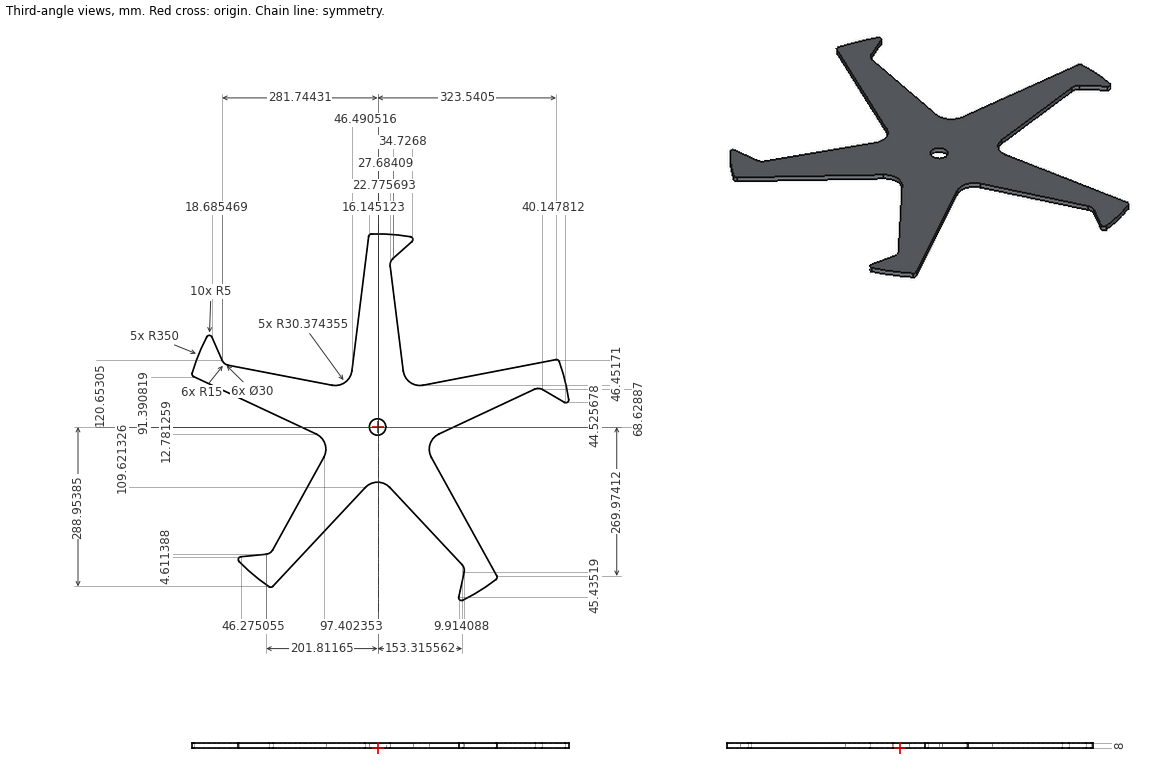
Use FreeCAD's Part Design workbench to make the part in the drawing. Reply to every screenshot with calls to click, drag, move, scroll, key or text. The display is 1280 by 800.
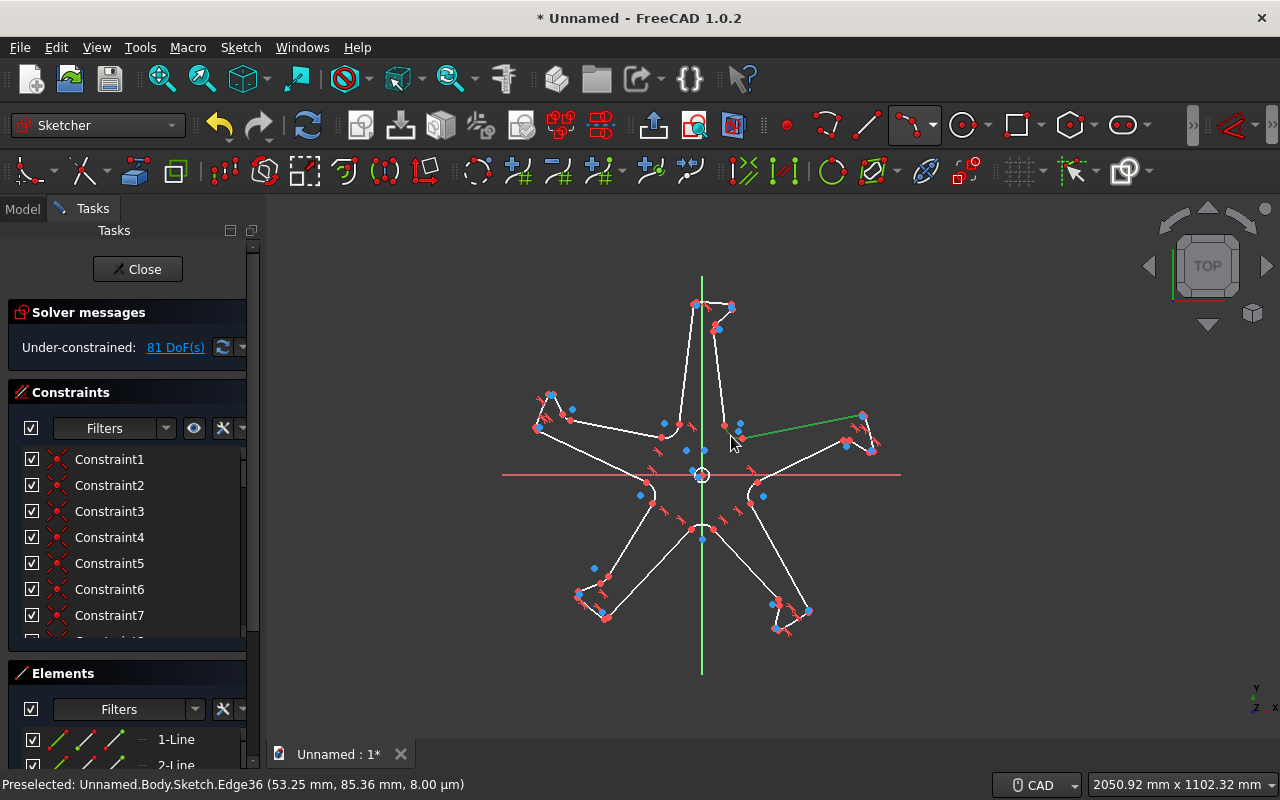
key(t)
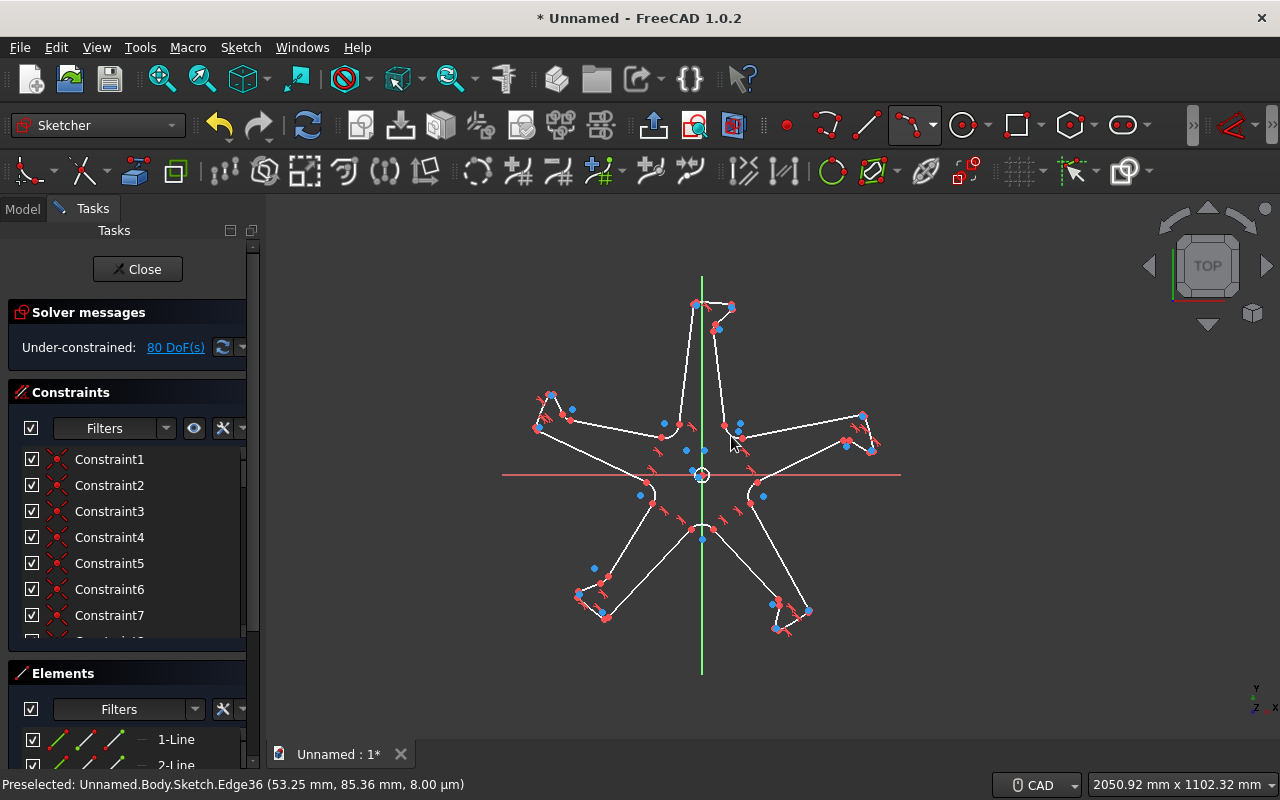
click(722, 397)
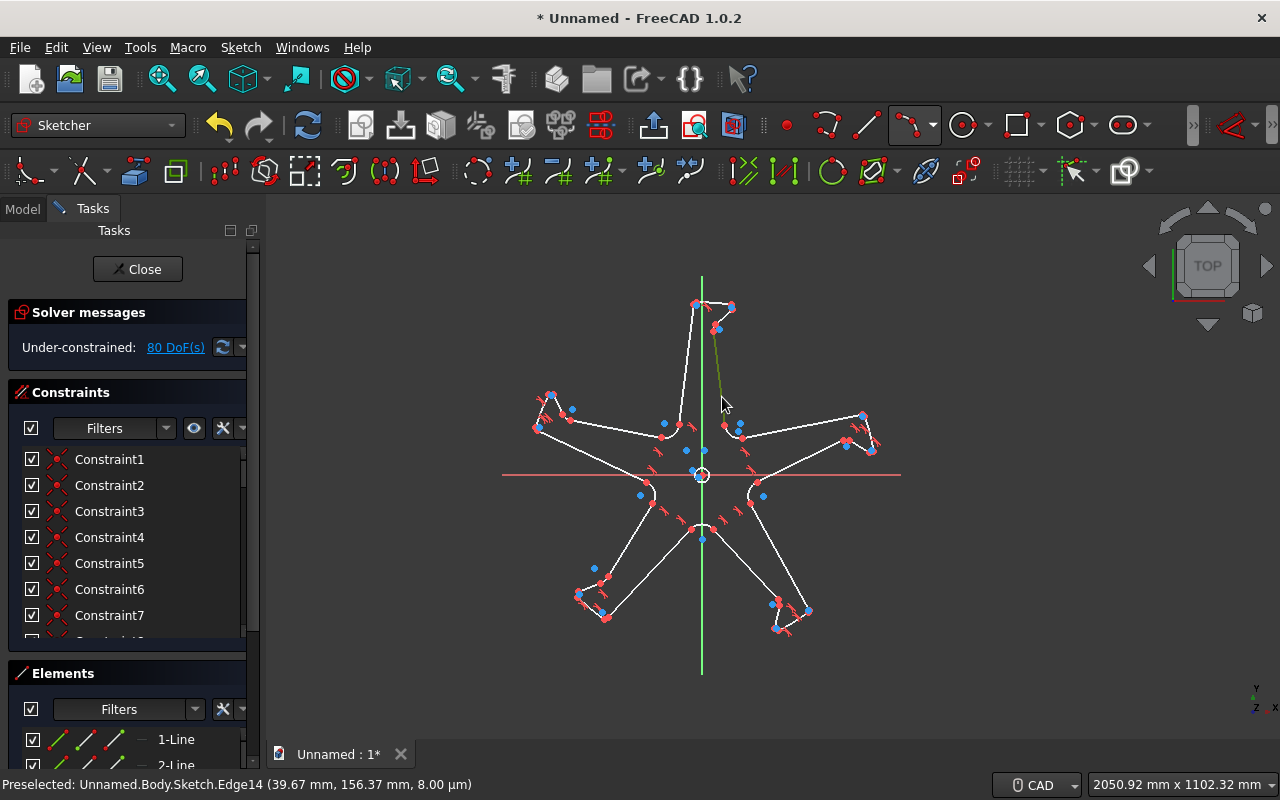
click(731, 436)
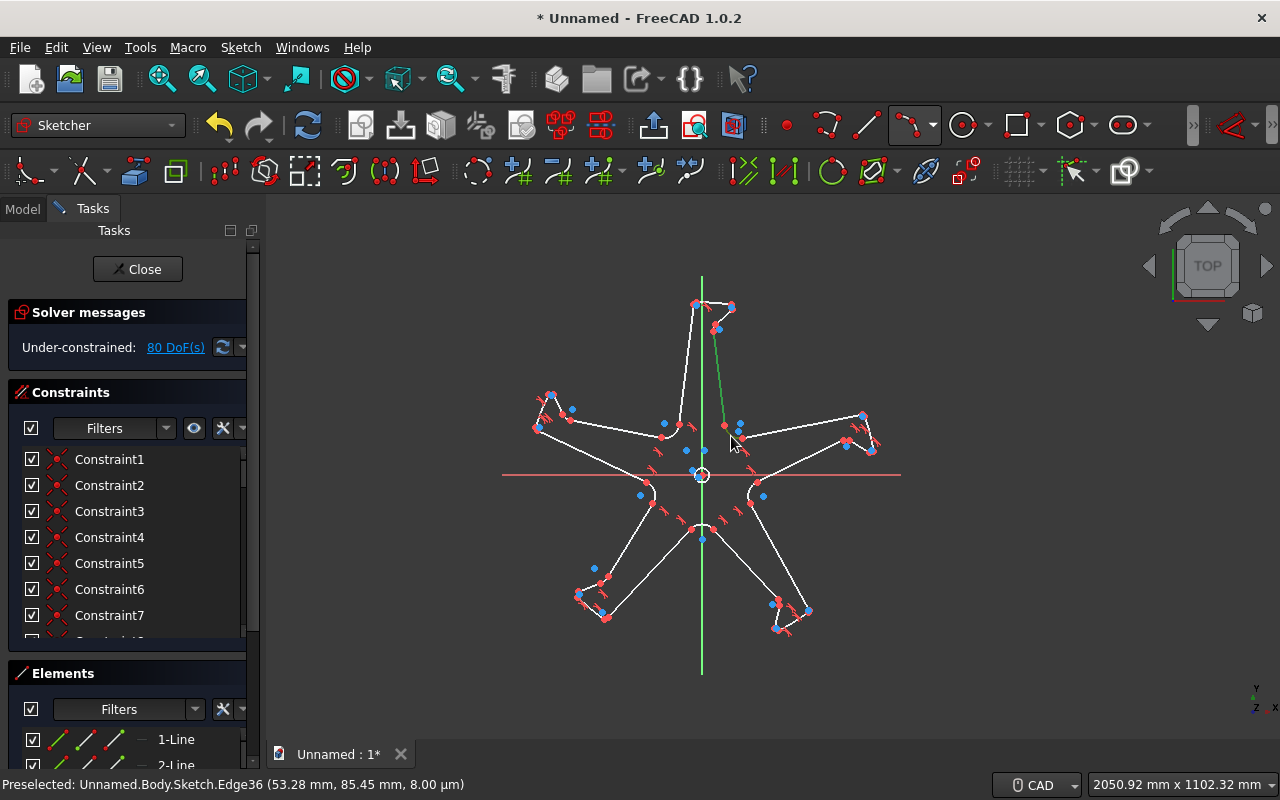
key(t)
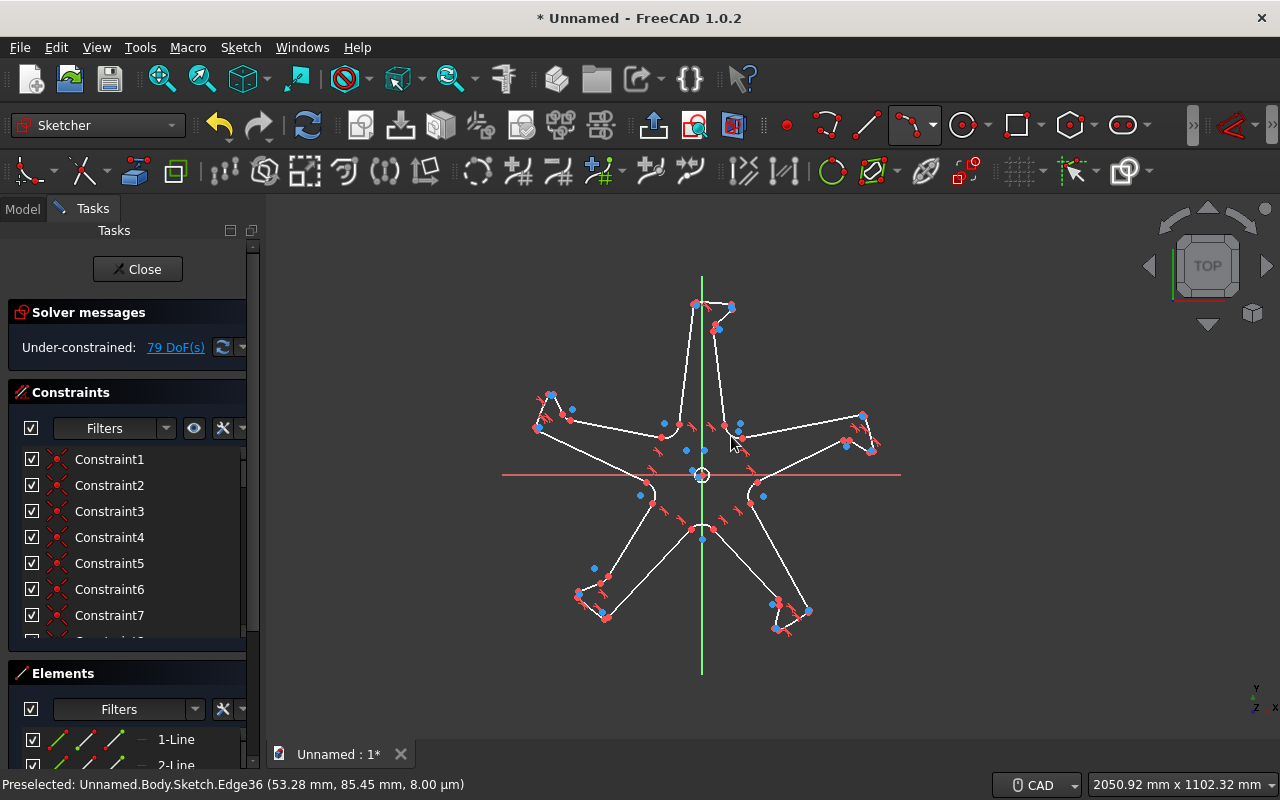
click(722, 397)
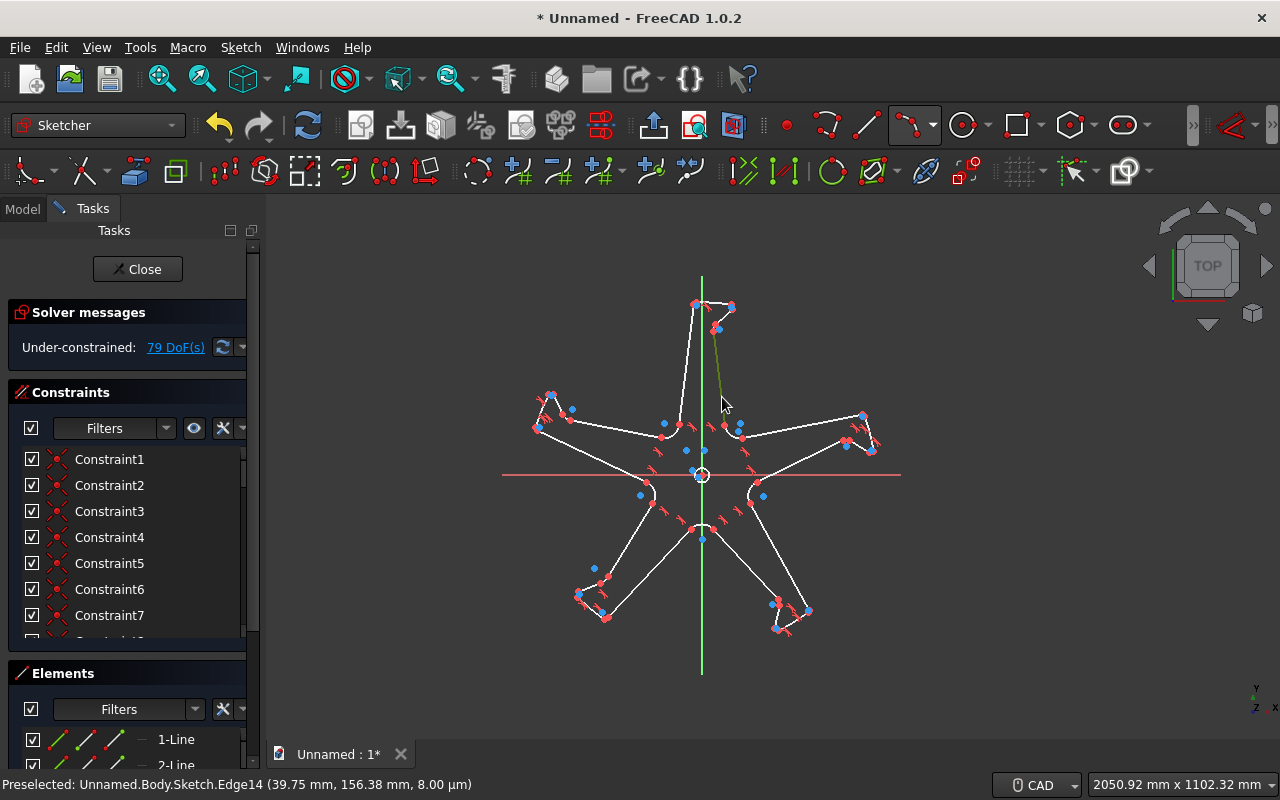
scroll(714, 328, up, 7)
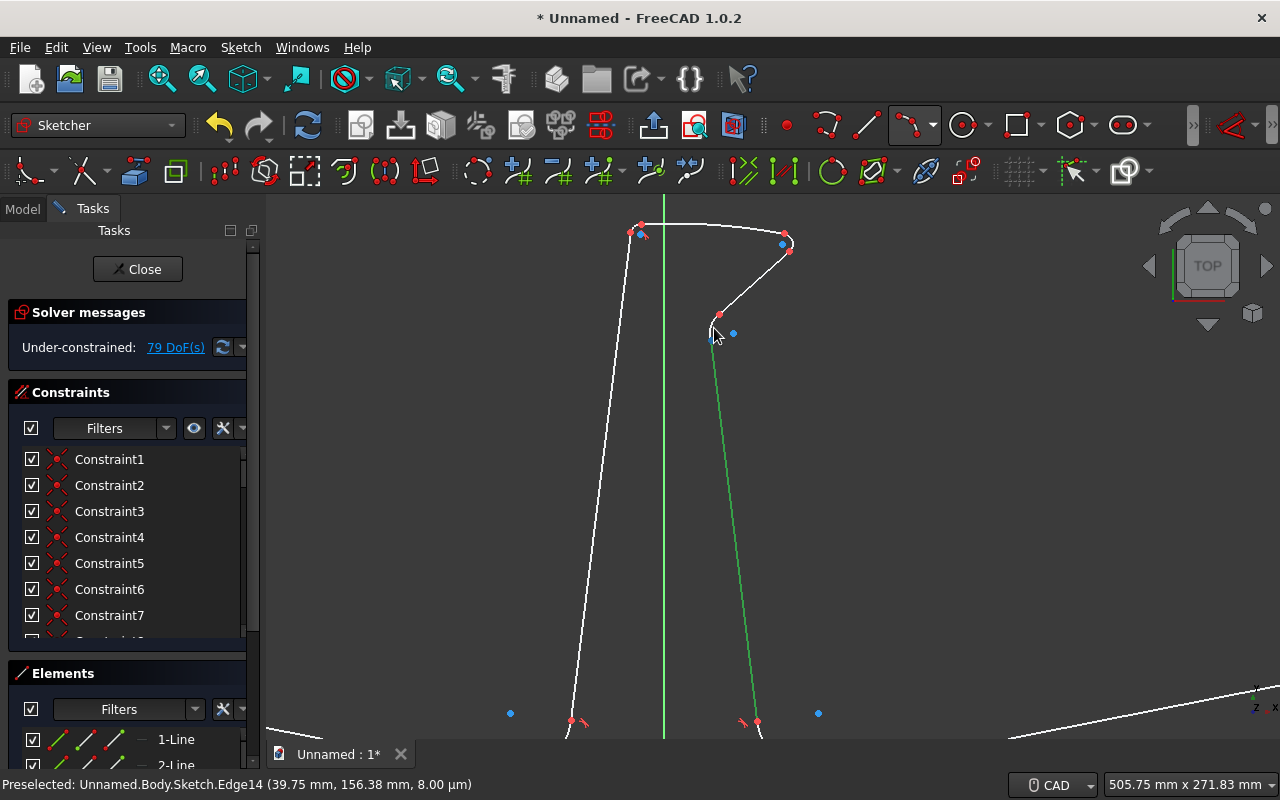
click(711, 326)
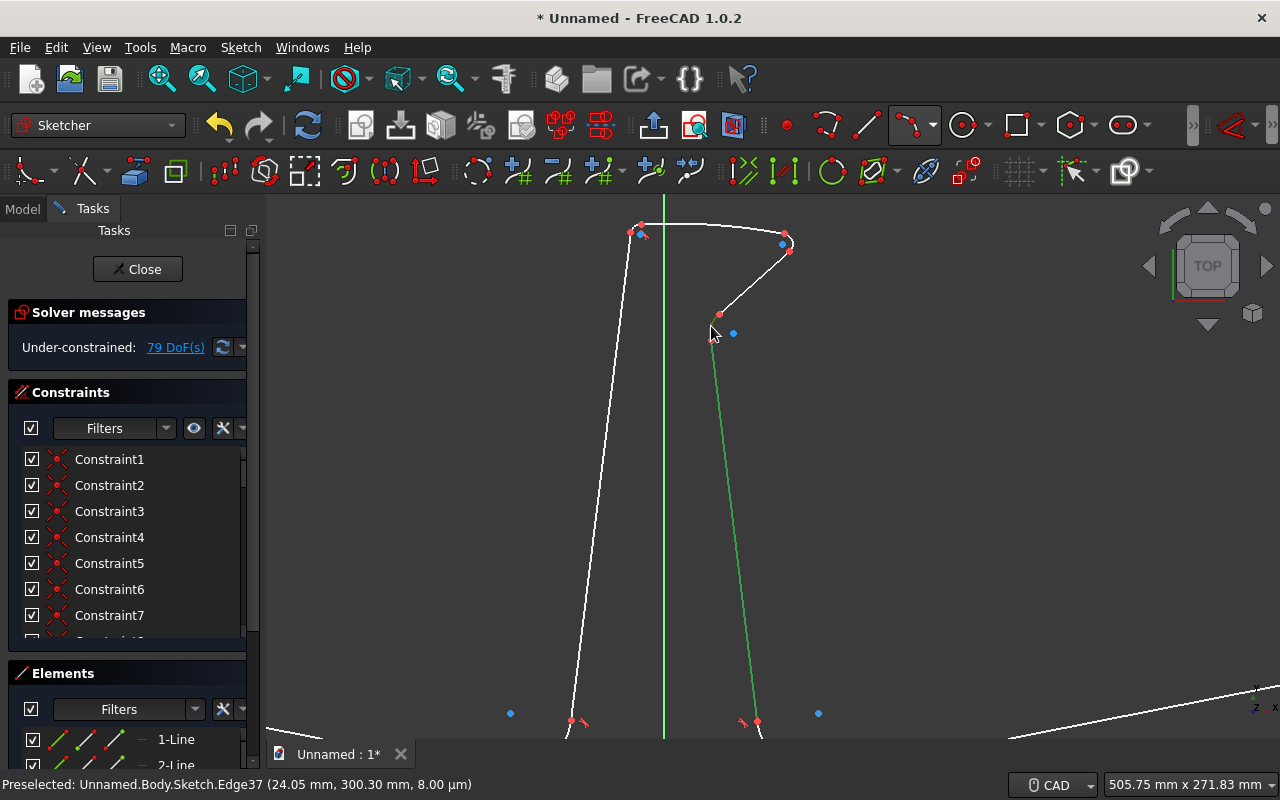
key(t)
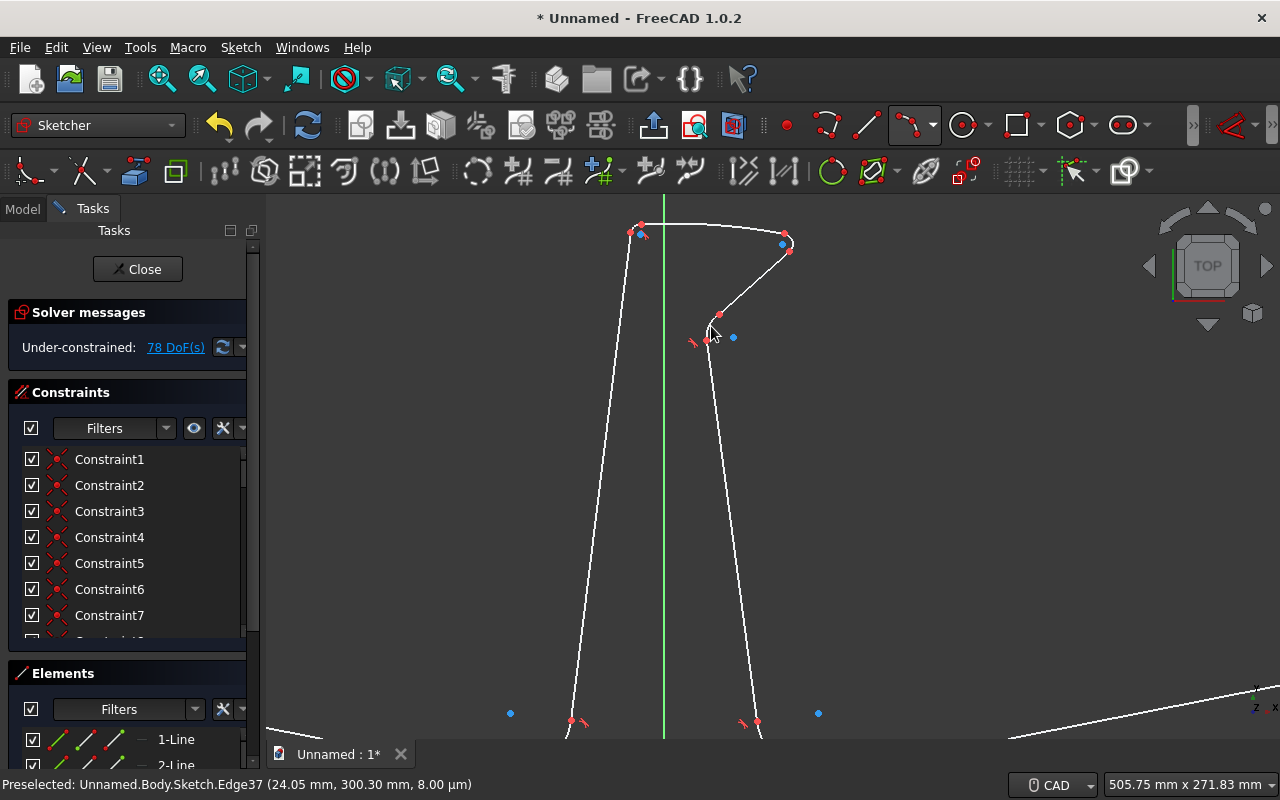
click(741, 295)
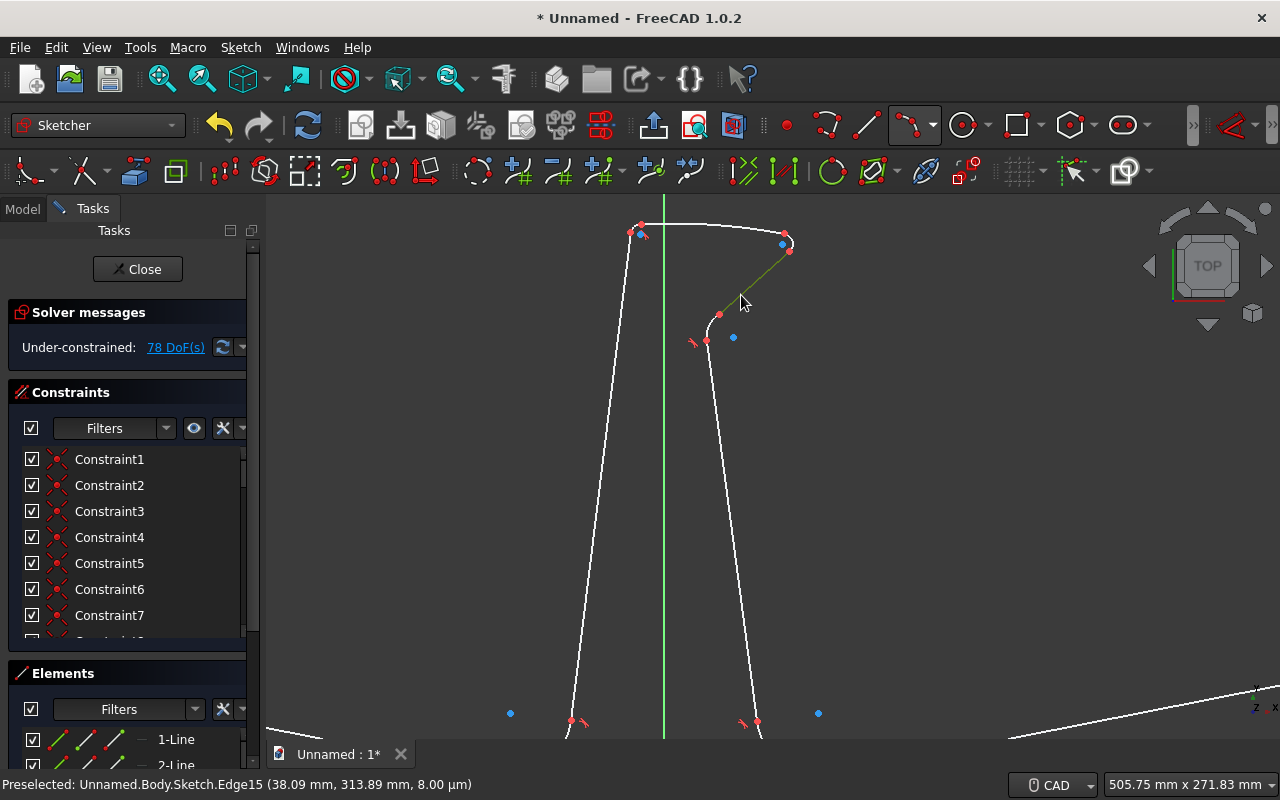
scroll(713, 320, up, 2)